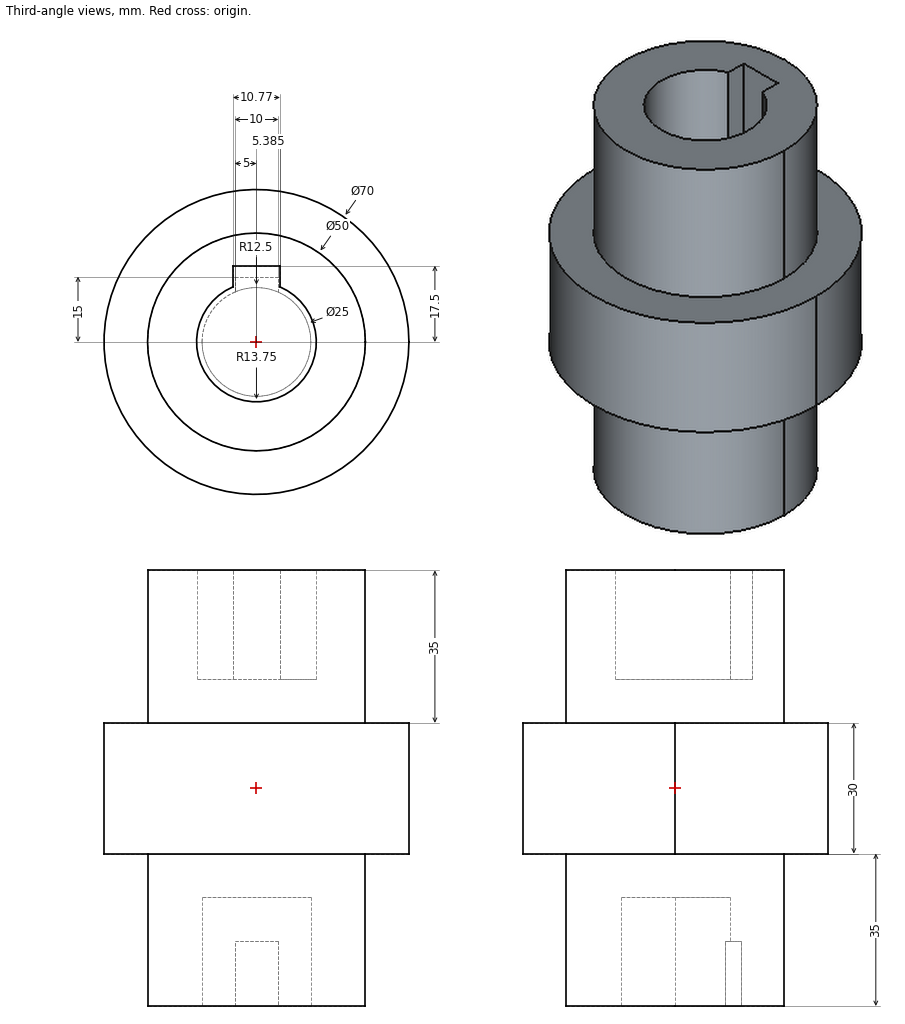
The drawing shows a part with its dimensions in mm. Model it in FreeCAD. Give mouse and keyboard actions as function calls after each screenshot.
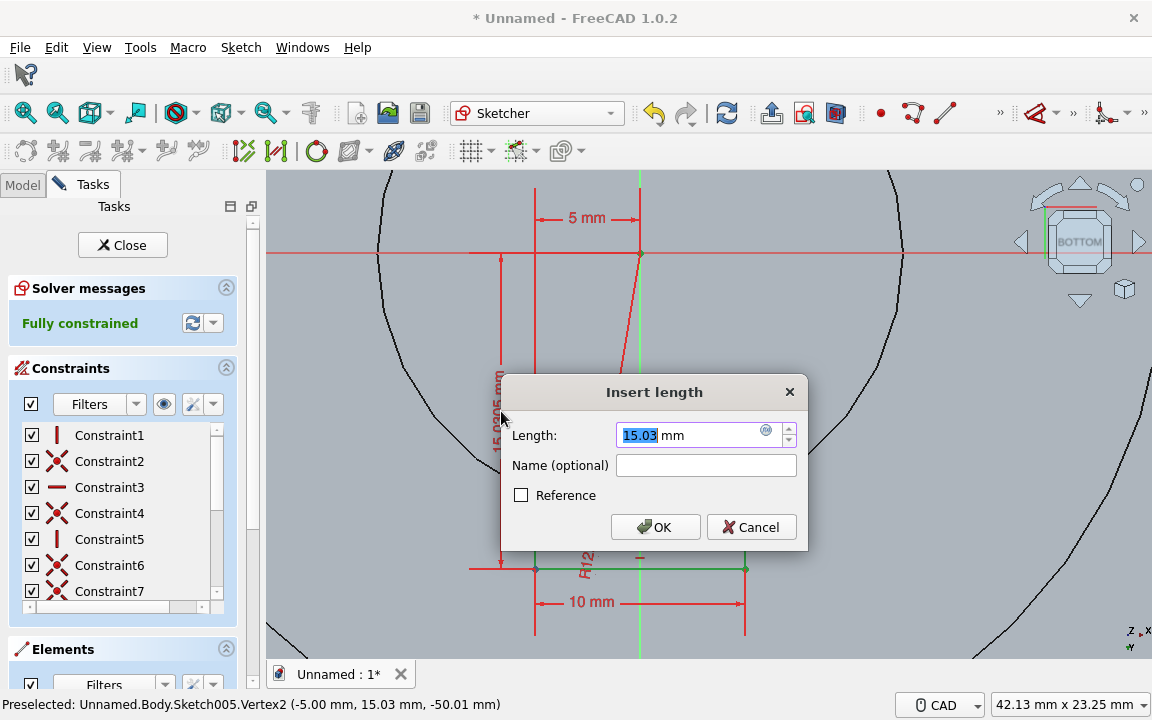
text(15)
key(Return)
key(Escape)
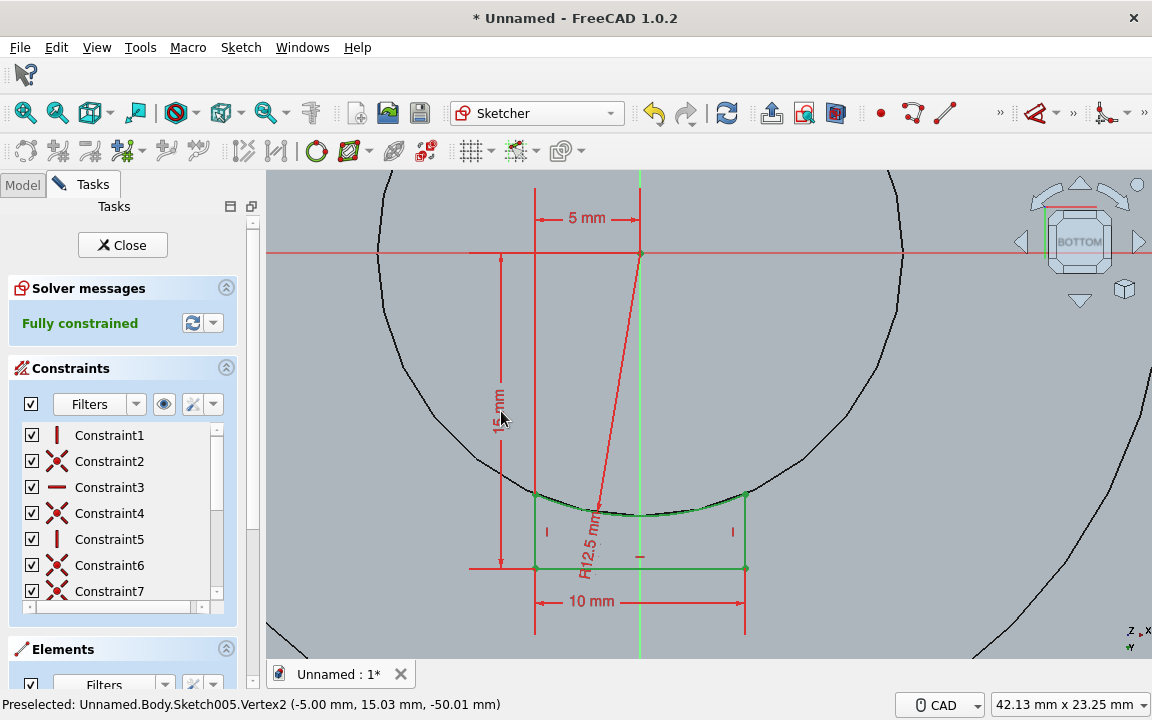
click(123, 245)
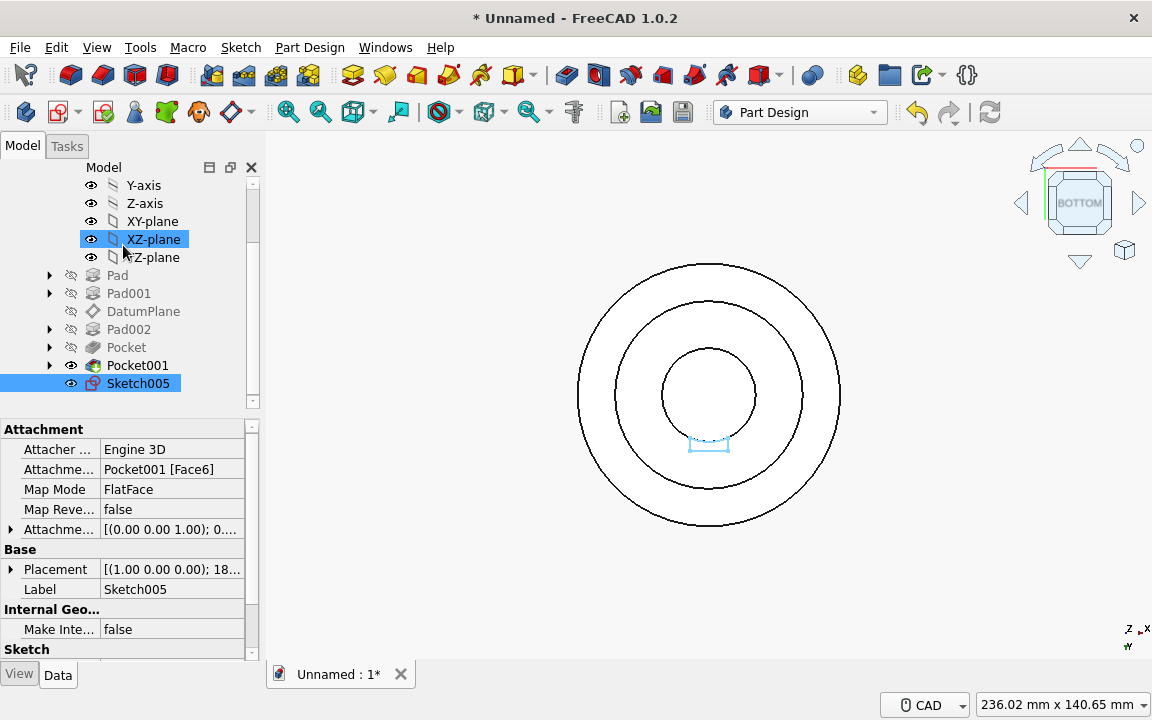
click(568, 76)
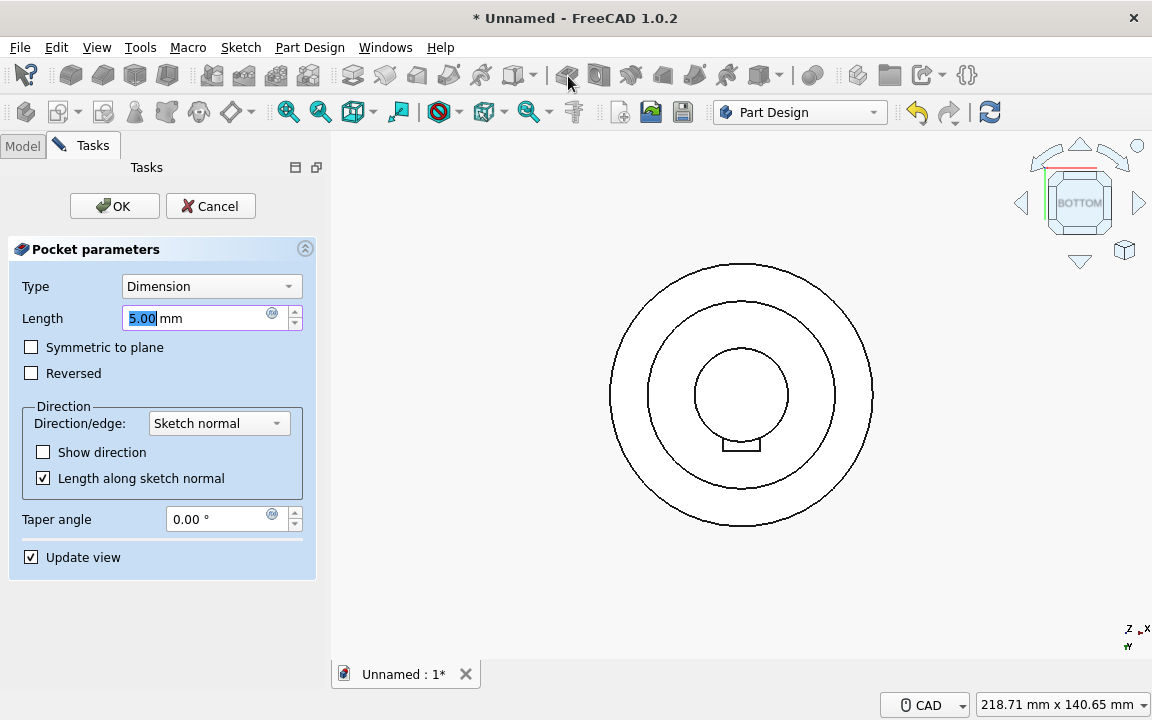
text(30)
key(Tab)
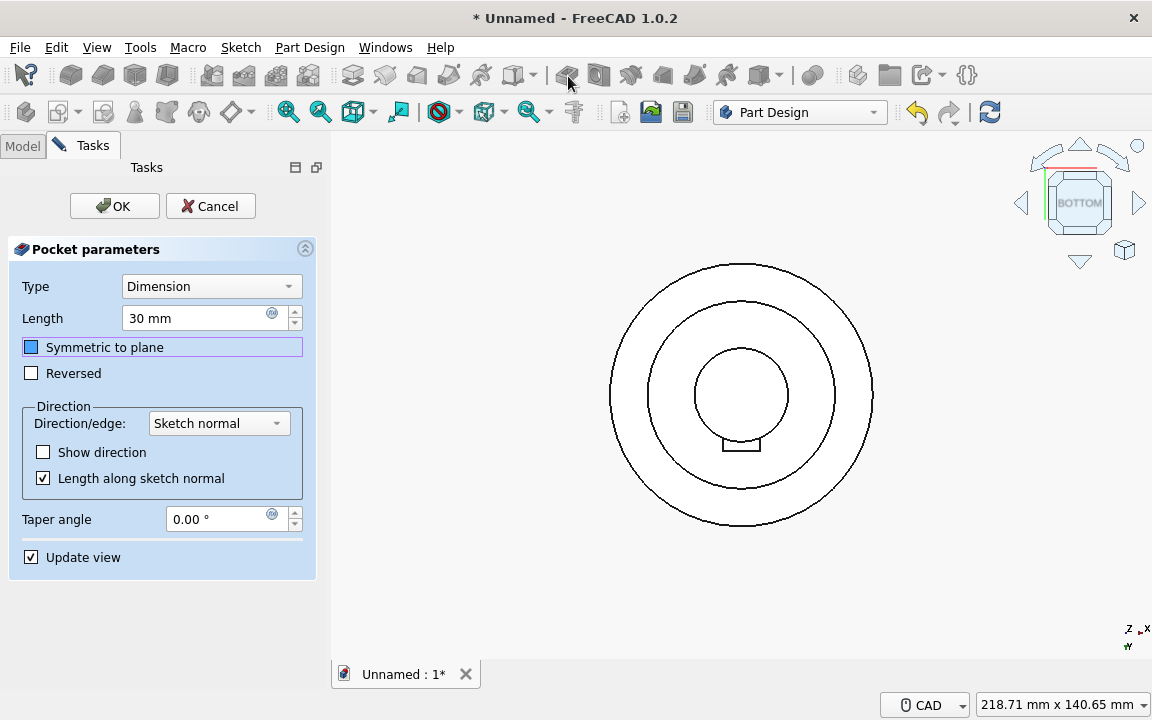
click(30, 347)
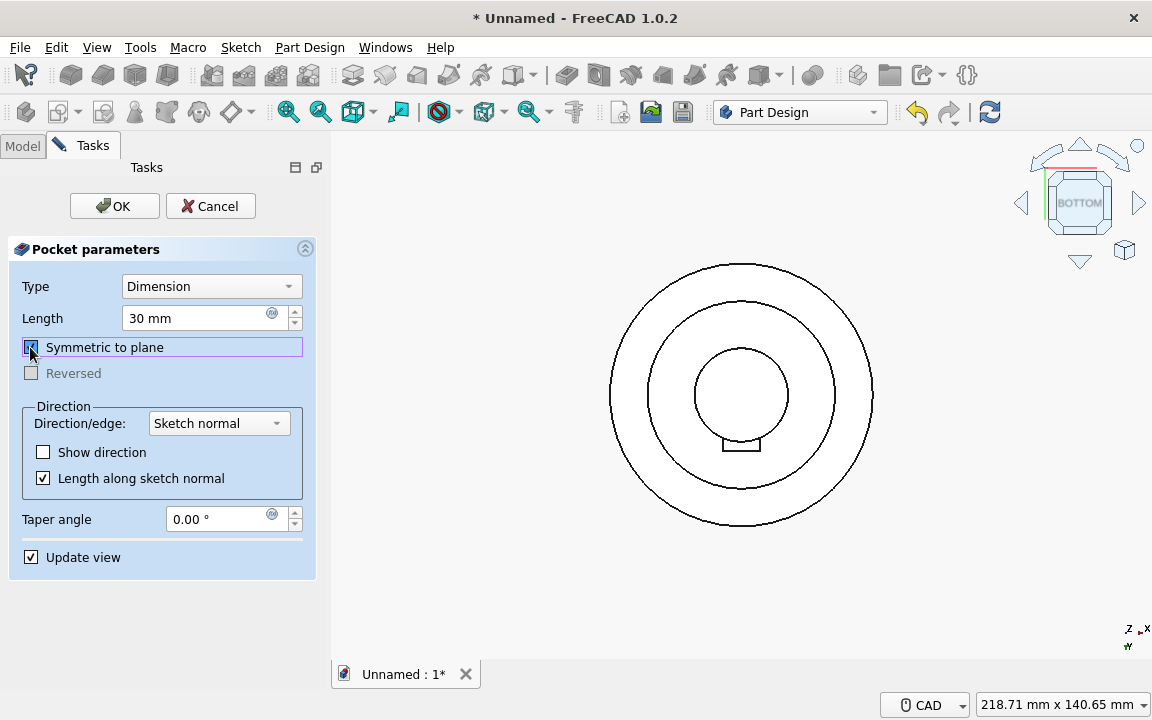
click(115, 206)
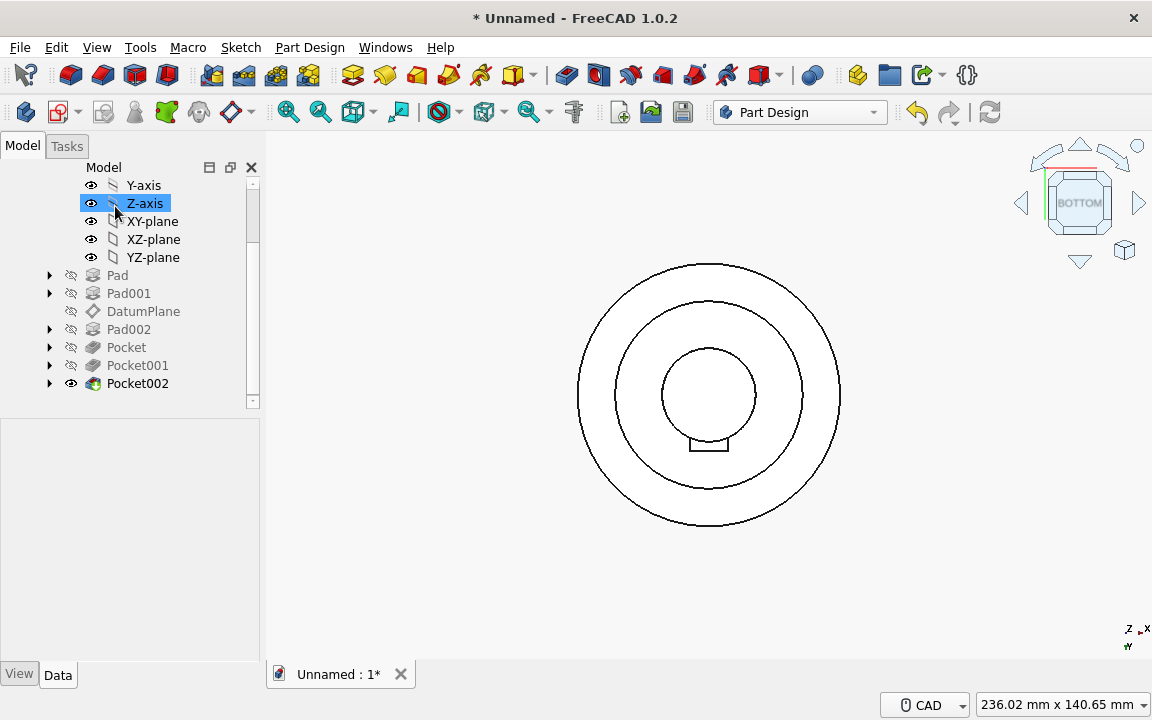
key(0)